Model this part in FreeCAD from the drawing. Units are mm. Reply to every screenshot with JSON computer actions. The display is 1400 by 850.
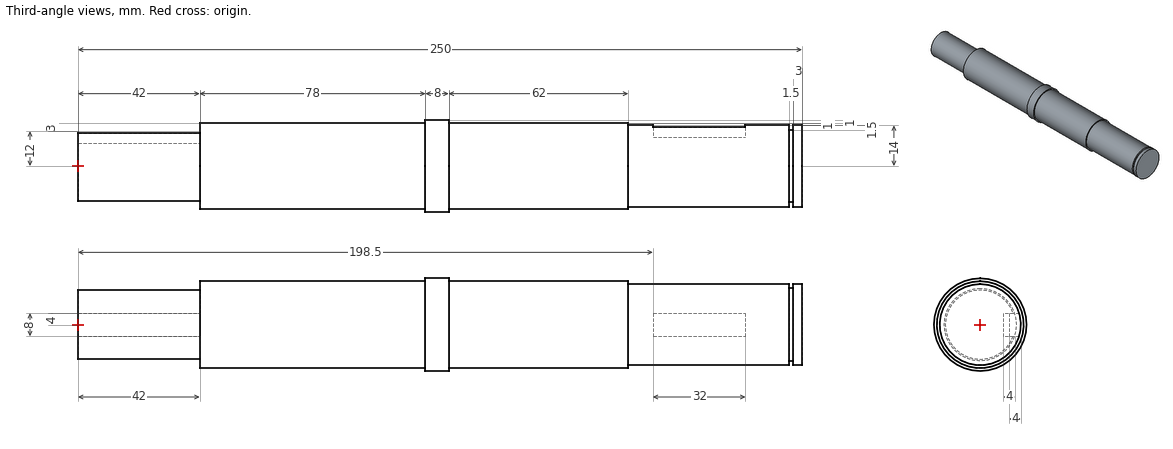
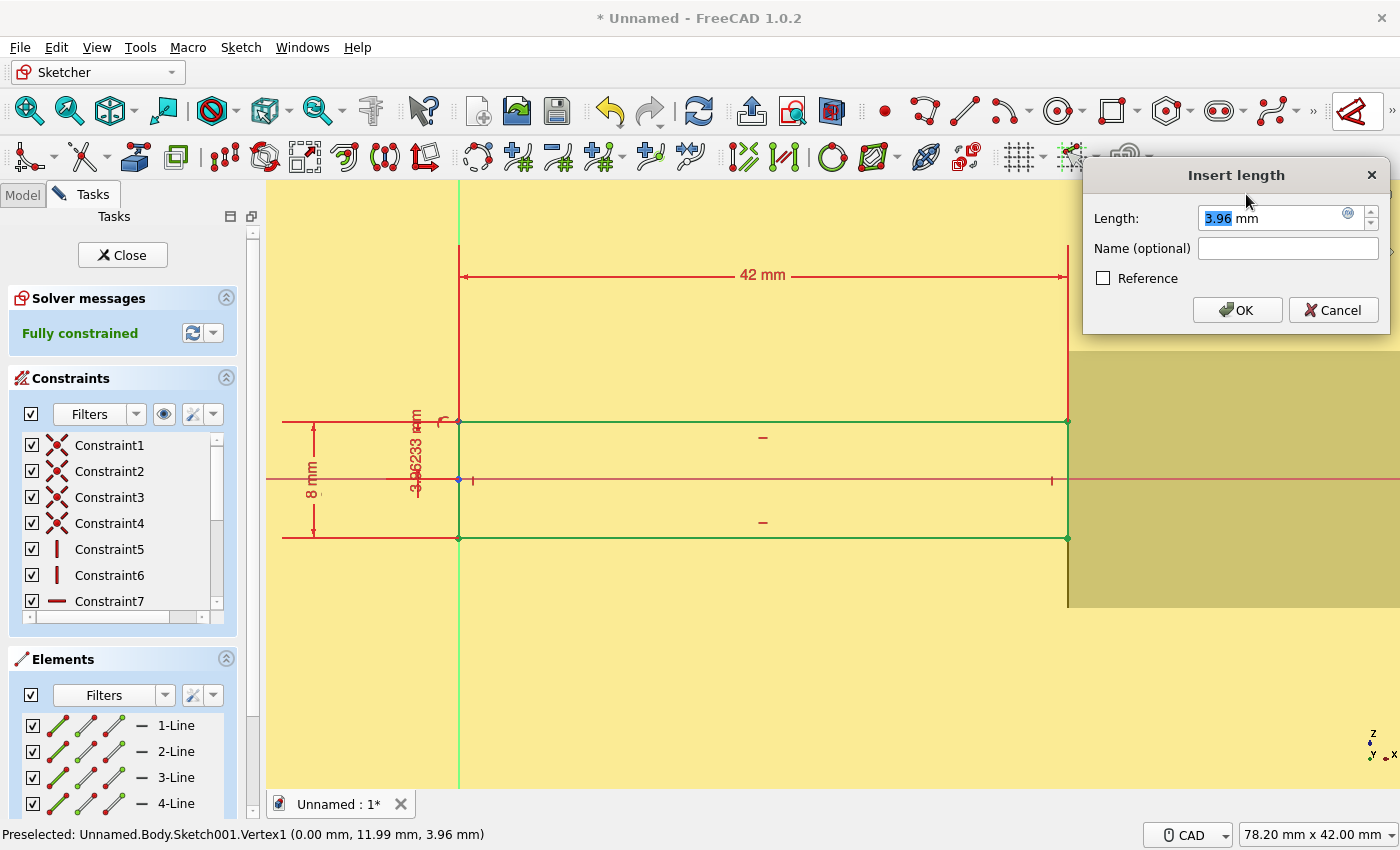
{"action": "type", "text": "4"}
{"action": "key", "text": "Return"}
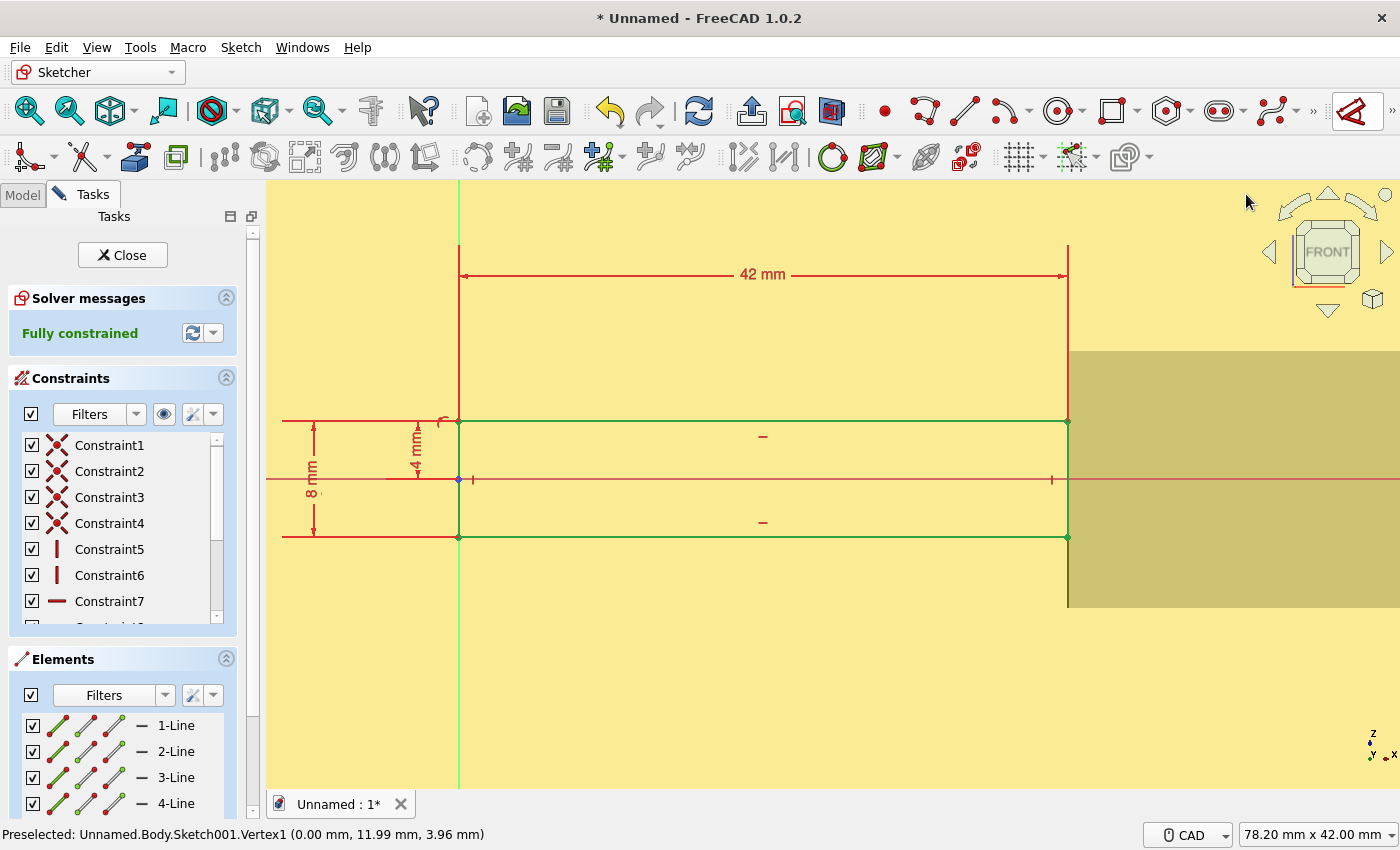
{"action": "left_click", "coordinate": [123, 255]}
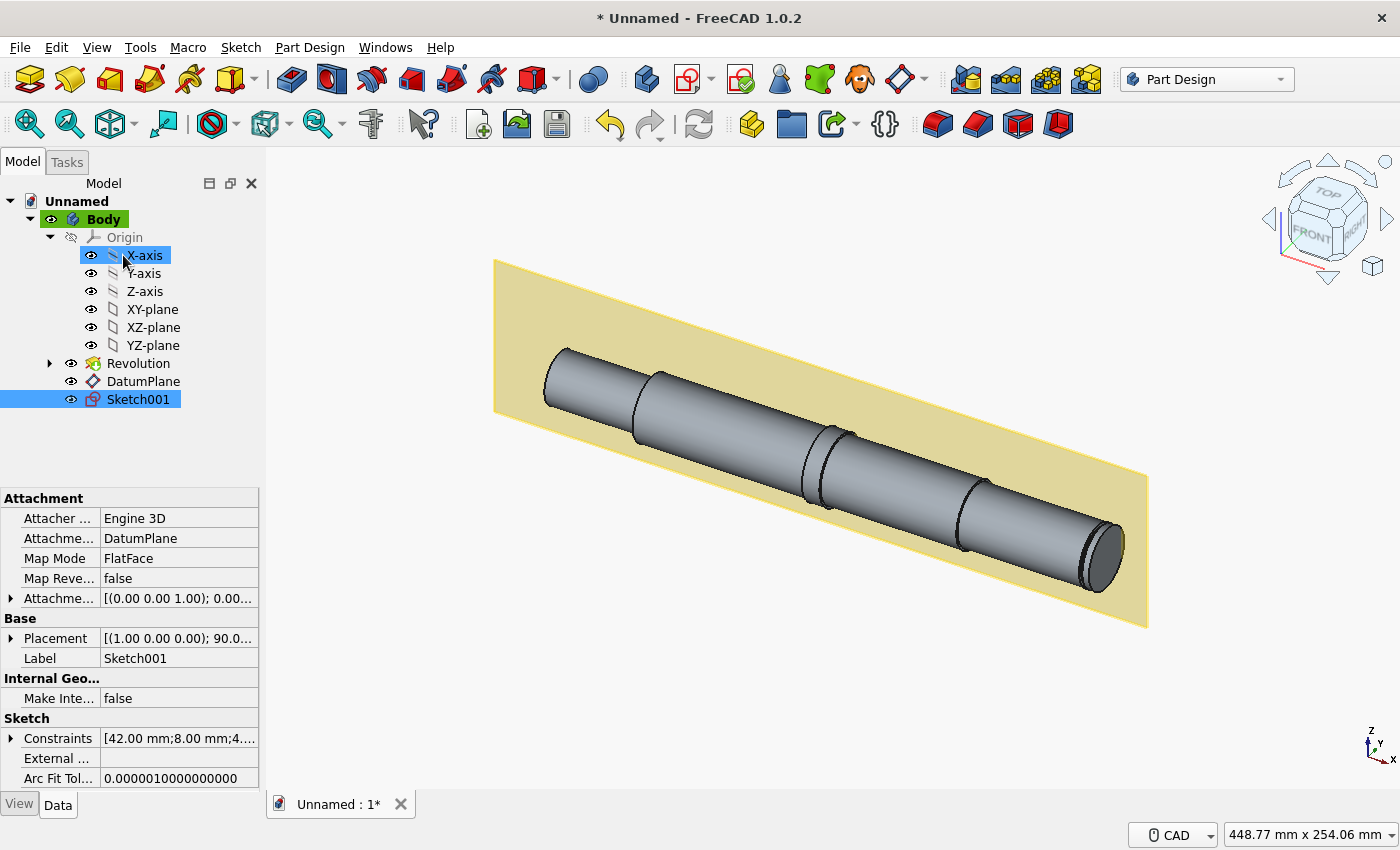
{"action": "left_click", "coordinate": [292, 80]}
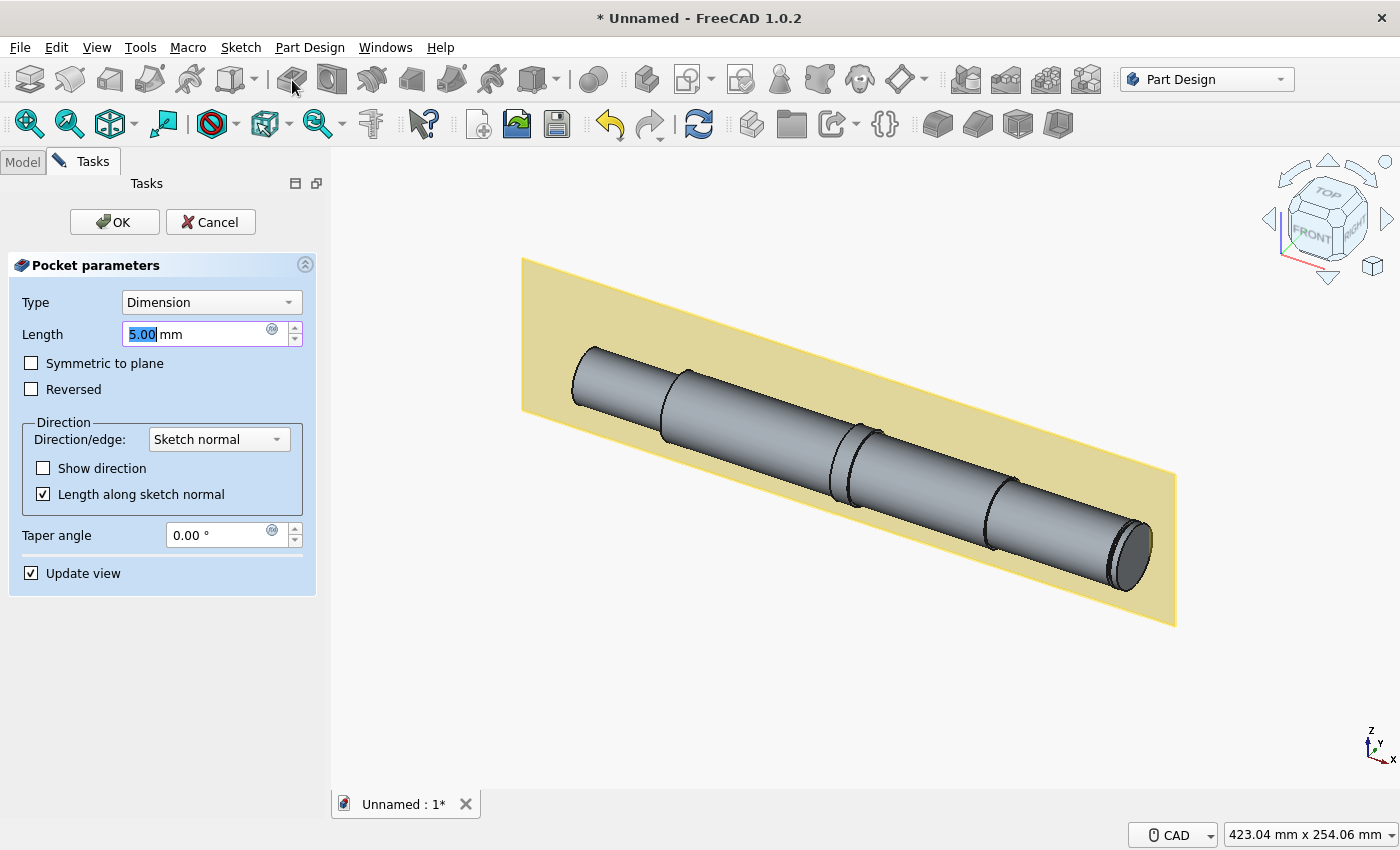
{"action": "type", "text": "4"}
{"action": "key", "text": "Tab"}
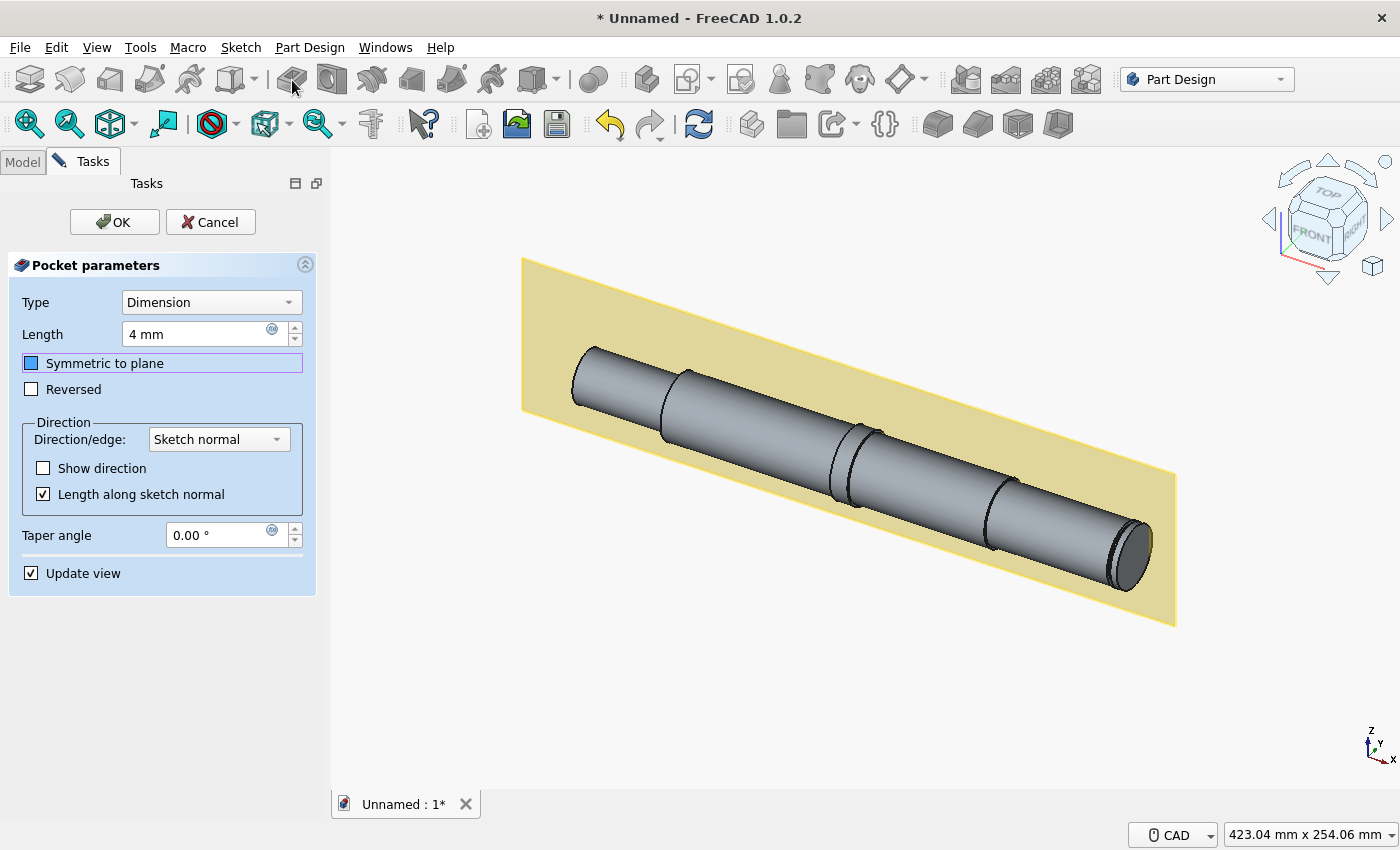
{"action": "left_click", "coordinate": [30, 389]}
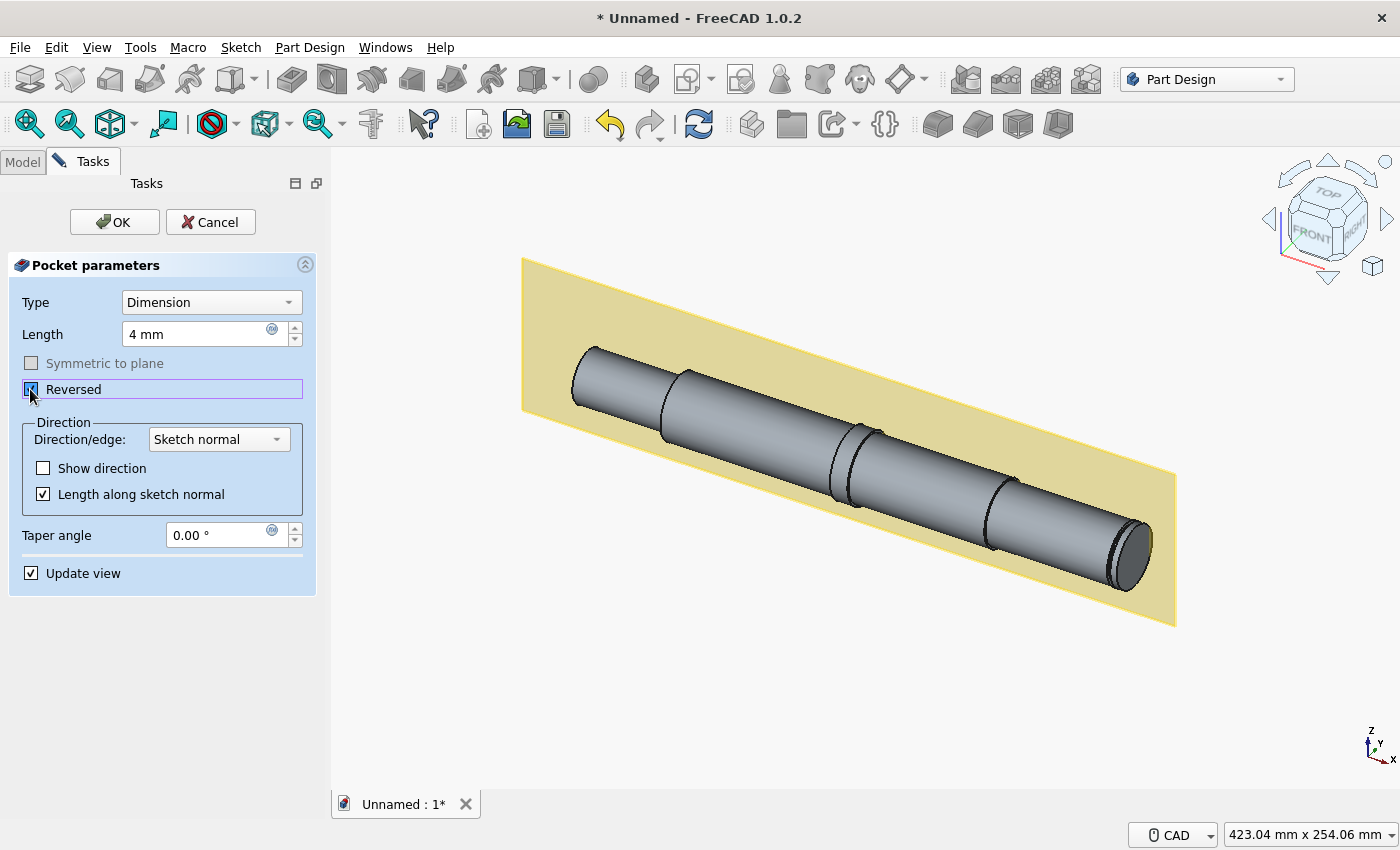
{"action": "left_click", "coordinate": [115, 222]}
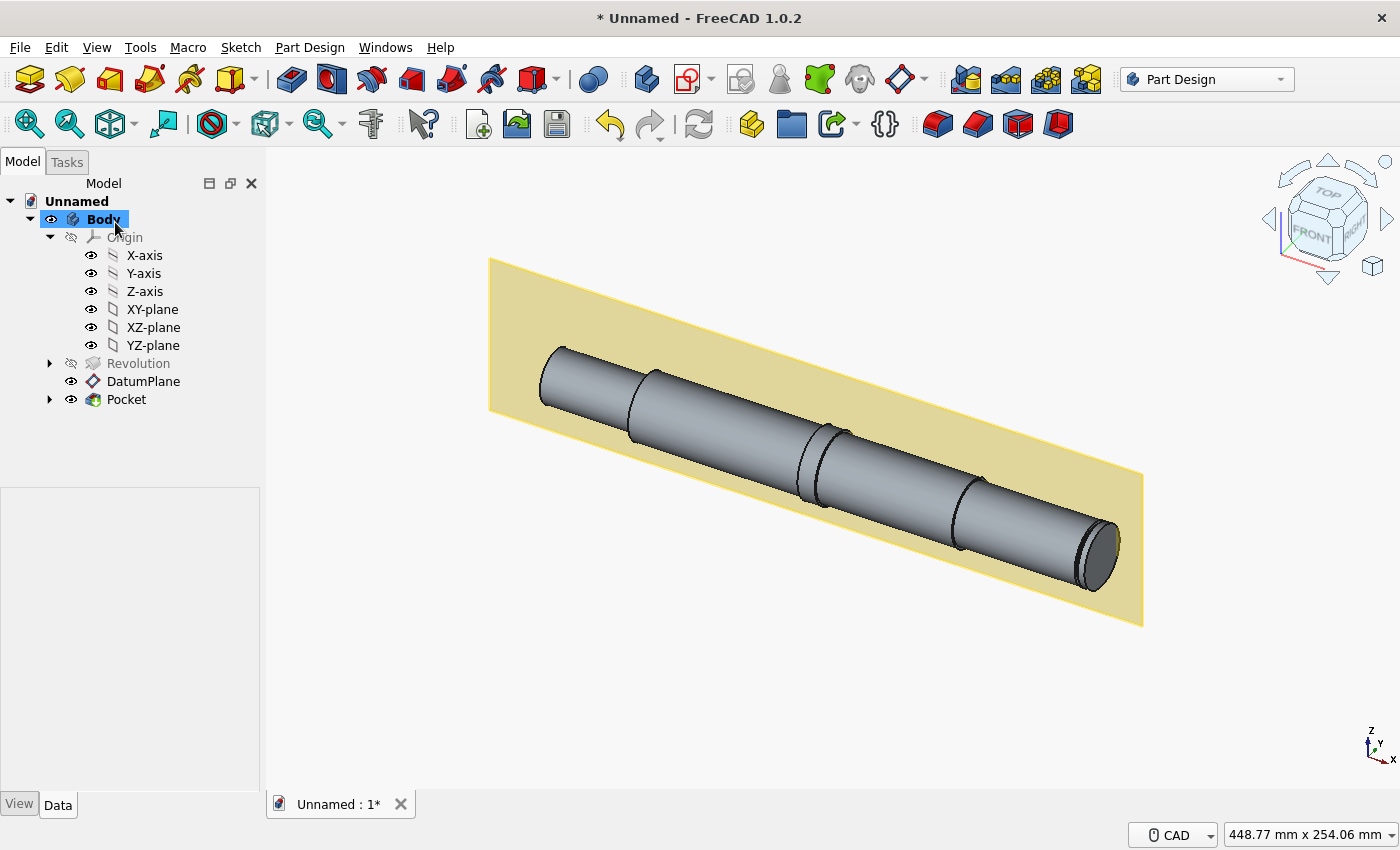
{"action": "left_click", "coordinate": [116, 381]}
{"action": "key", "text": "space"}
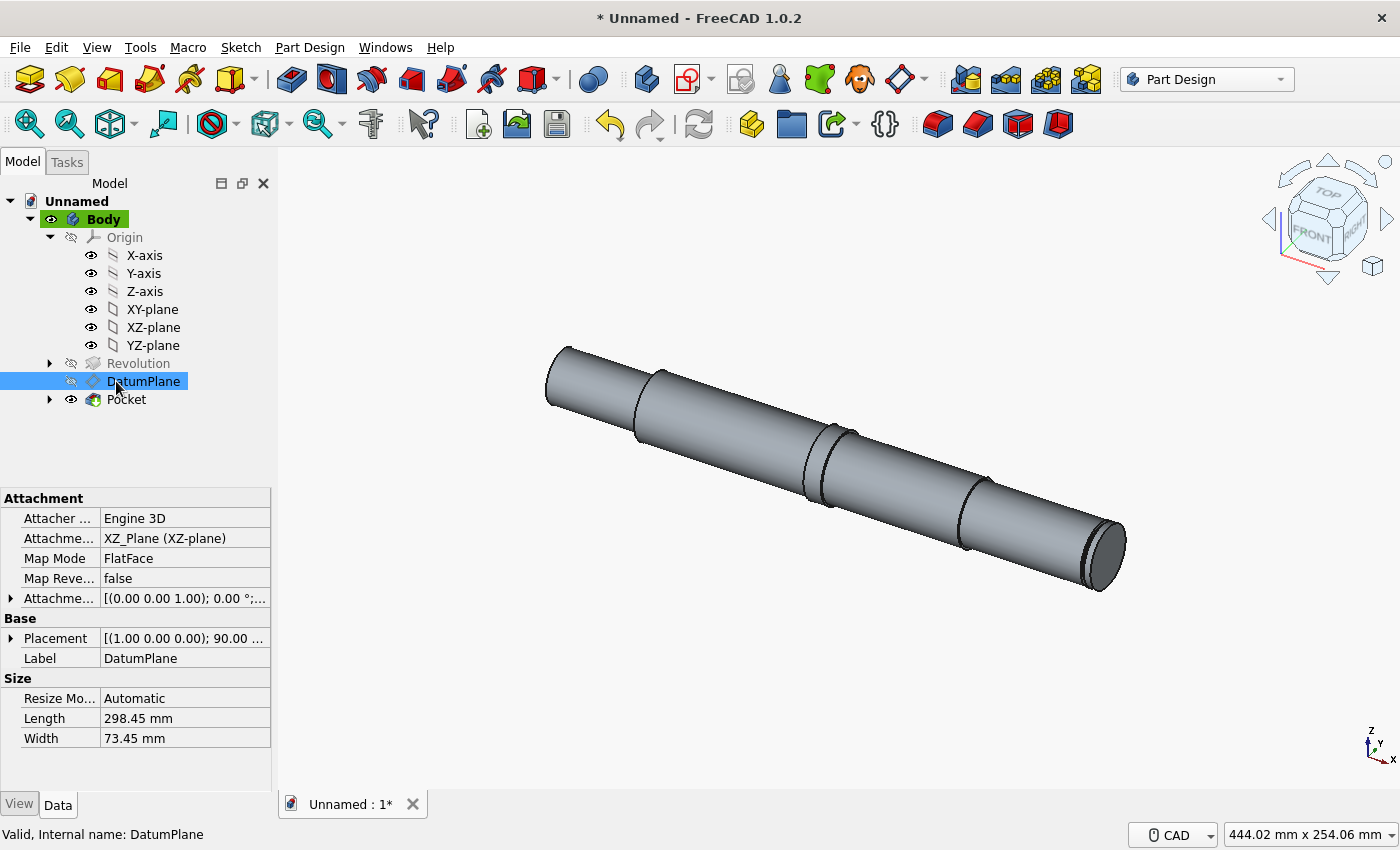
{"action": "left_click", "coordinate": [136, 327]}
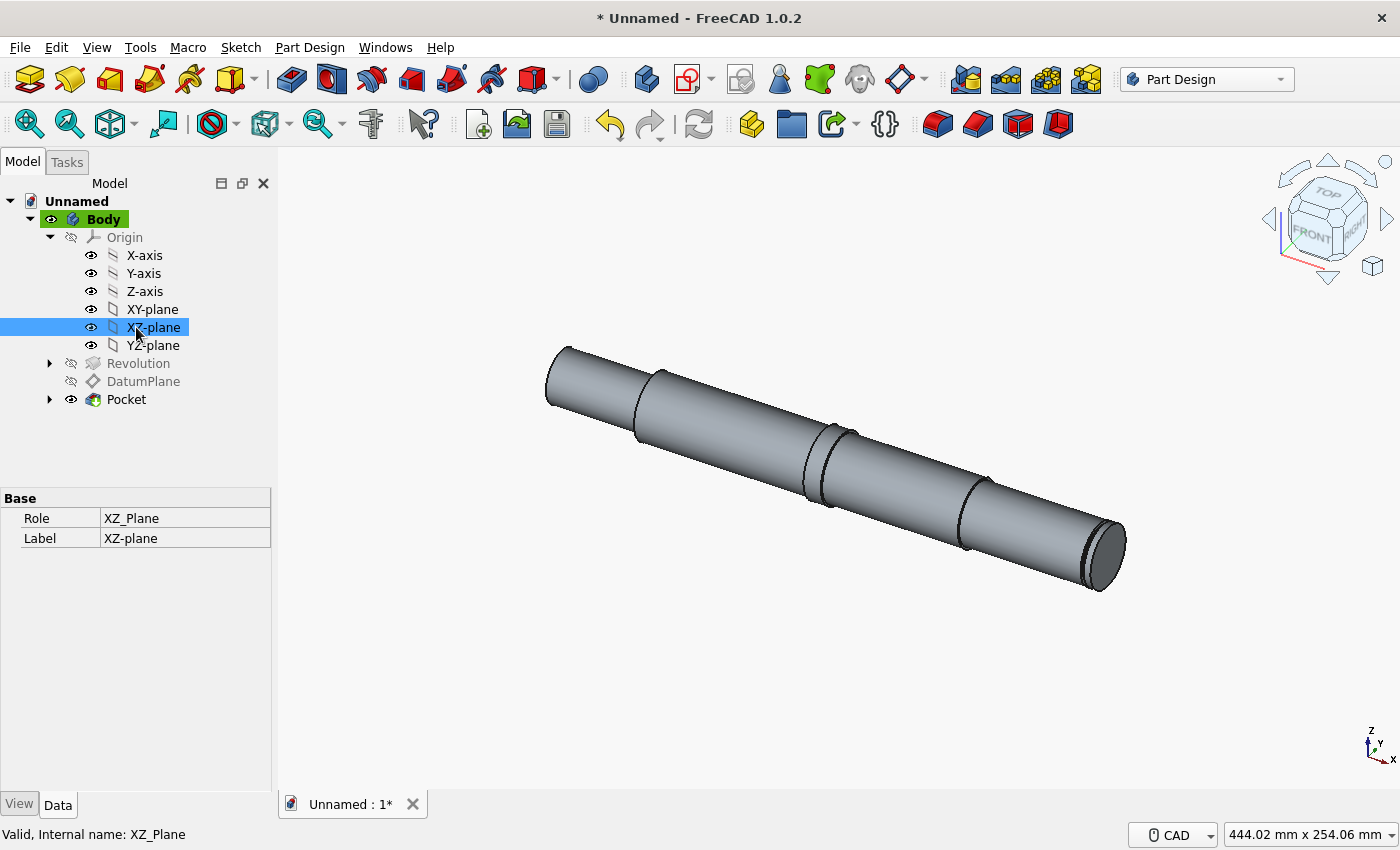
{"action": "left_click", "coordinate": [900, 80]}